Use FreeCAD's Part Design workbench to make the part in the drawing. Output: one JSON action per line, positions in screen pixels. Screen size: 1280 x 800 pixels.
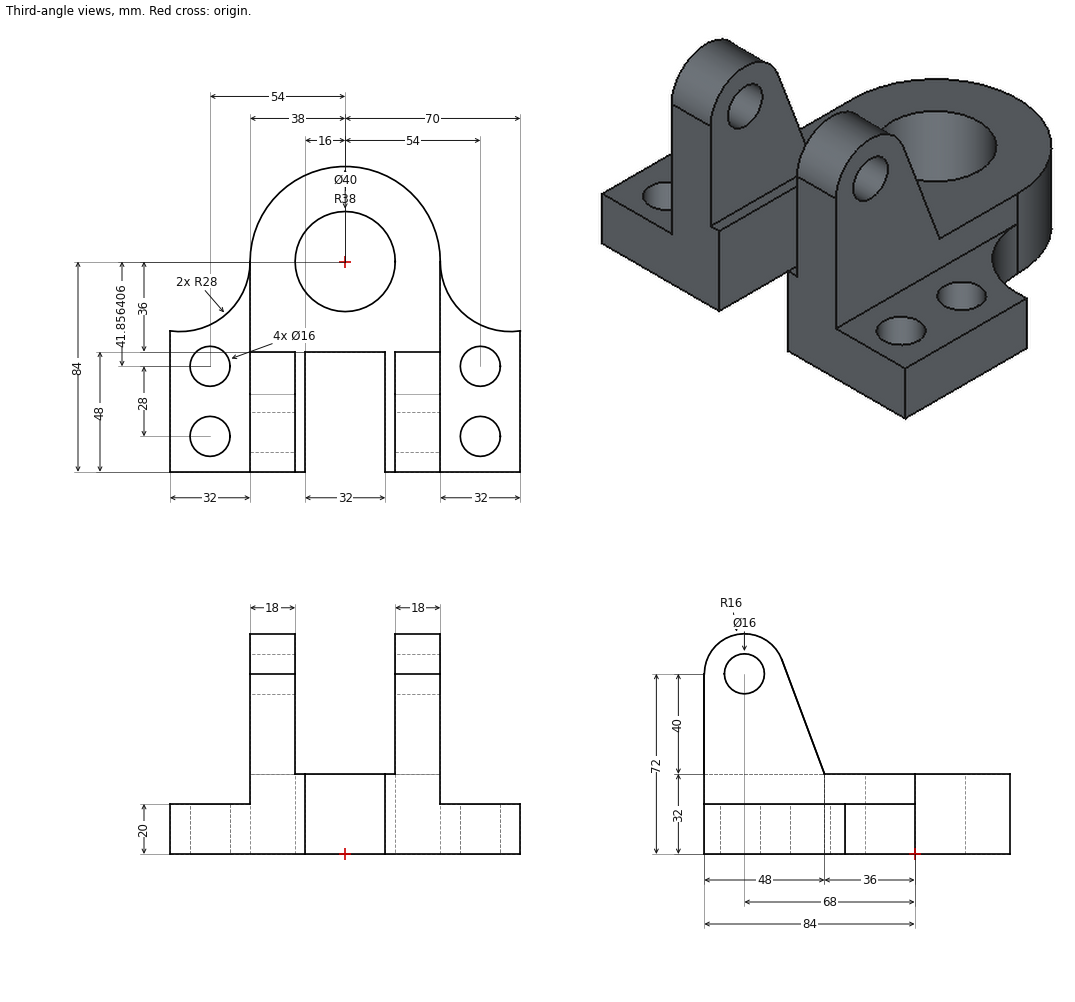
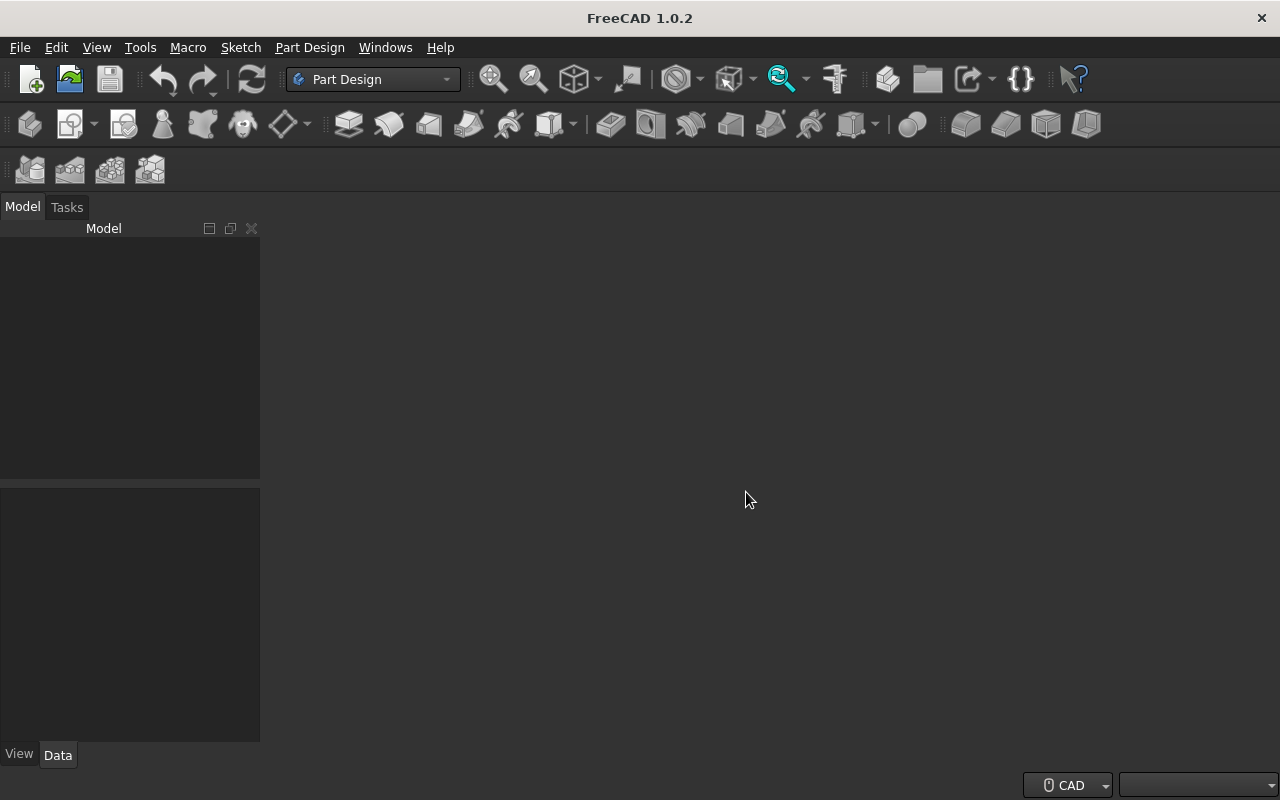
{"action": "left_click", "coordinate": [30, 80]}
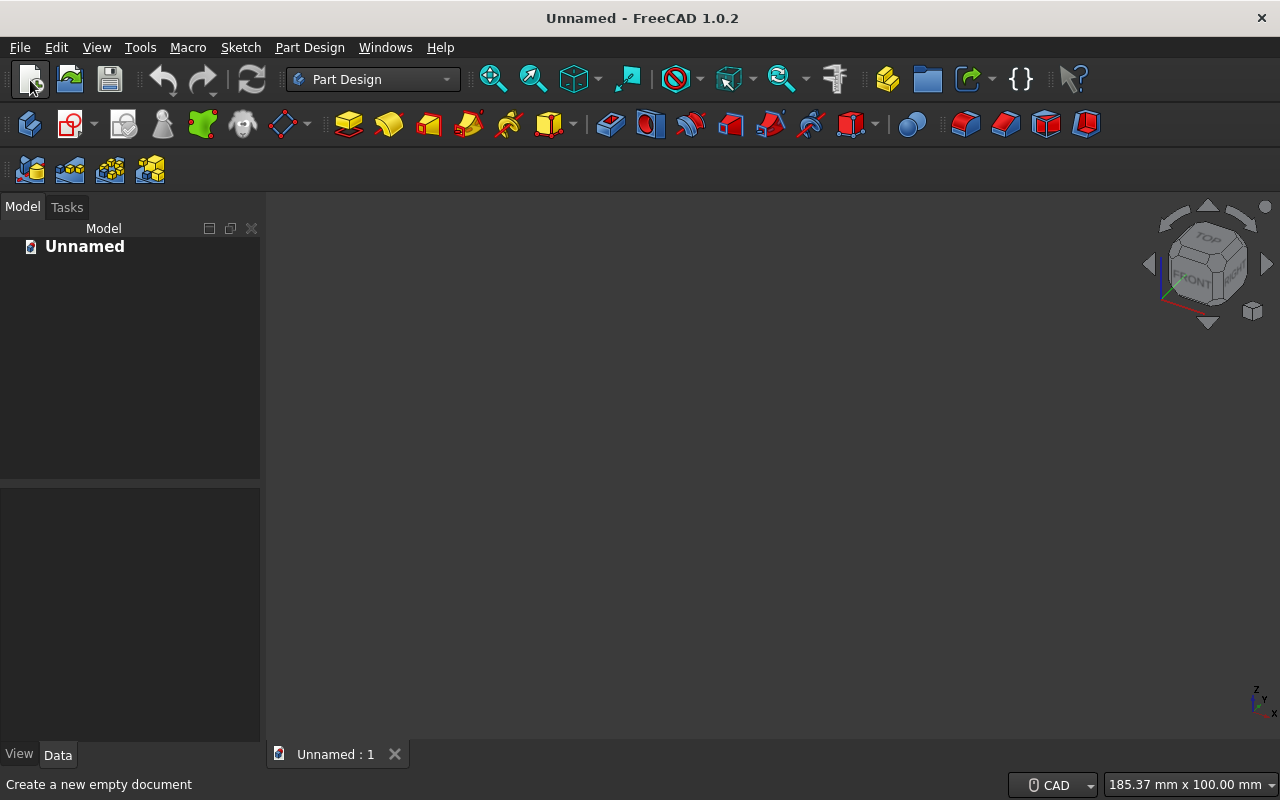
{"action": "left_click", "coordinate": [70, 124]}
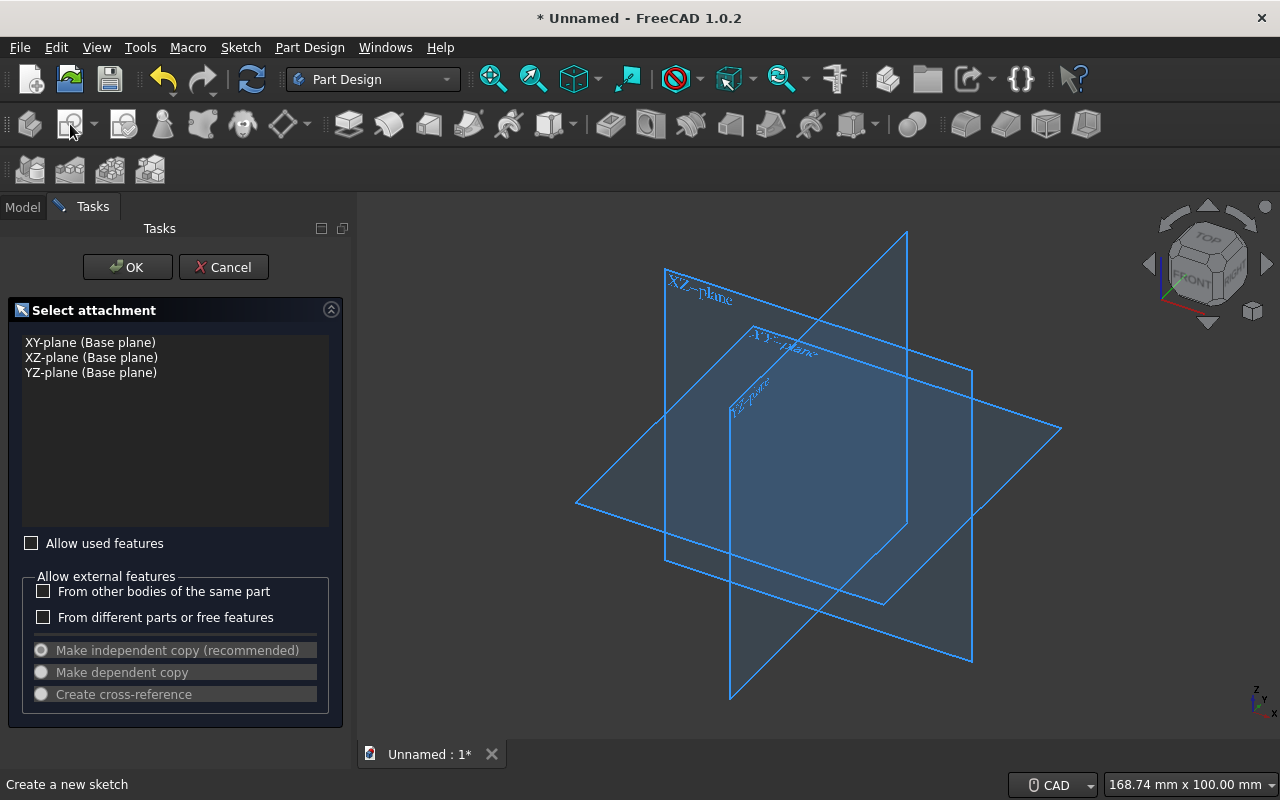
{"action": "left_click", "coordinate": [82, 342]}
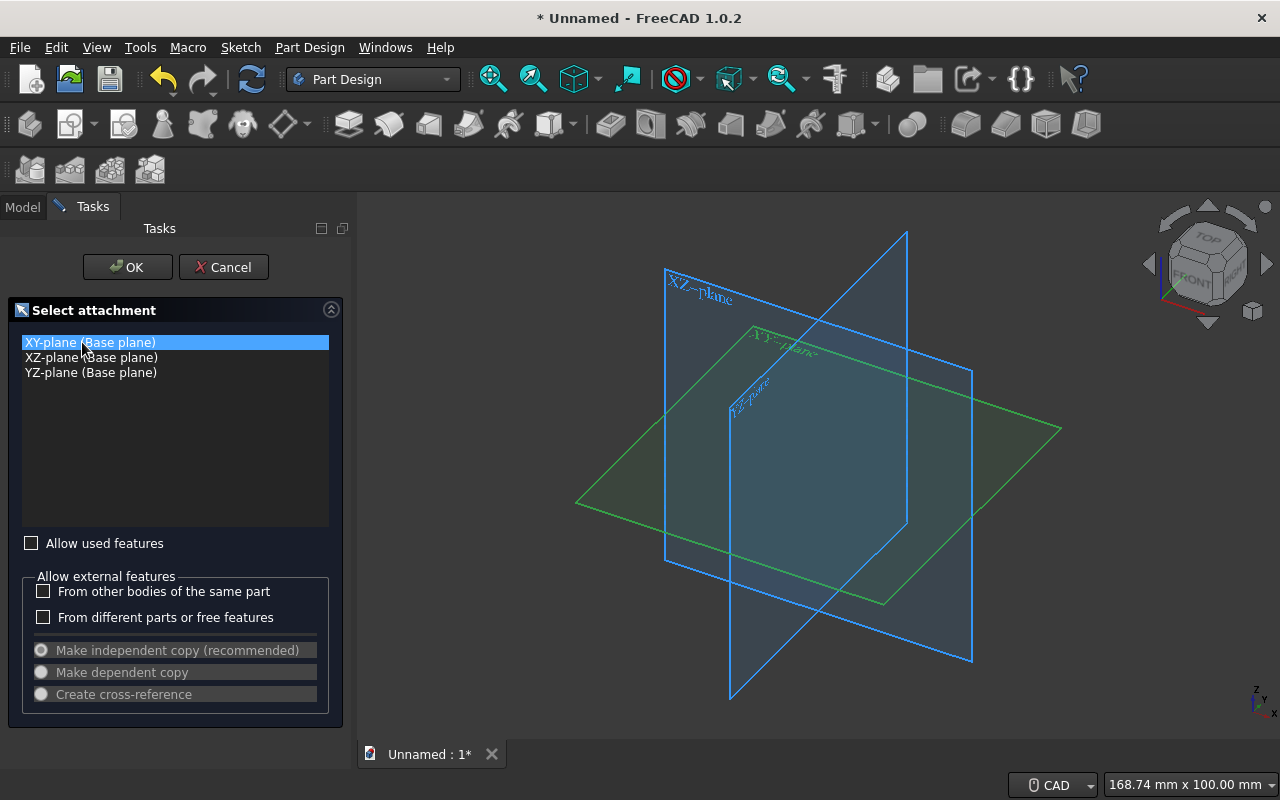
{"action": "left_click", "coordinate": [128, 267]}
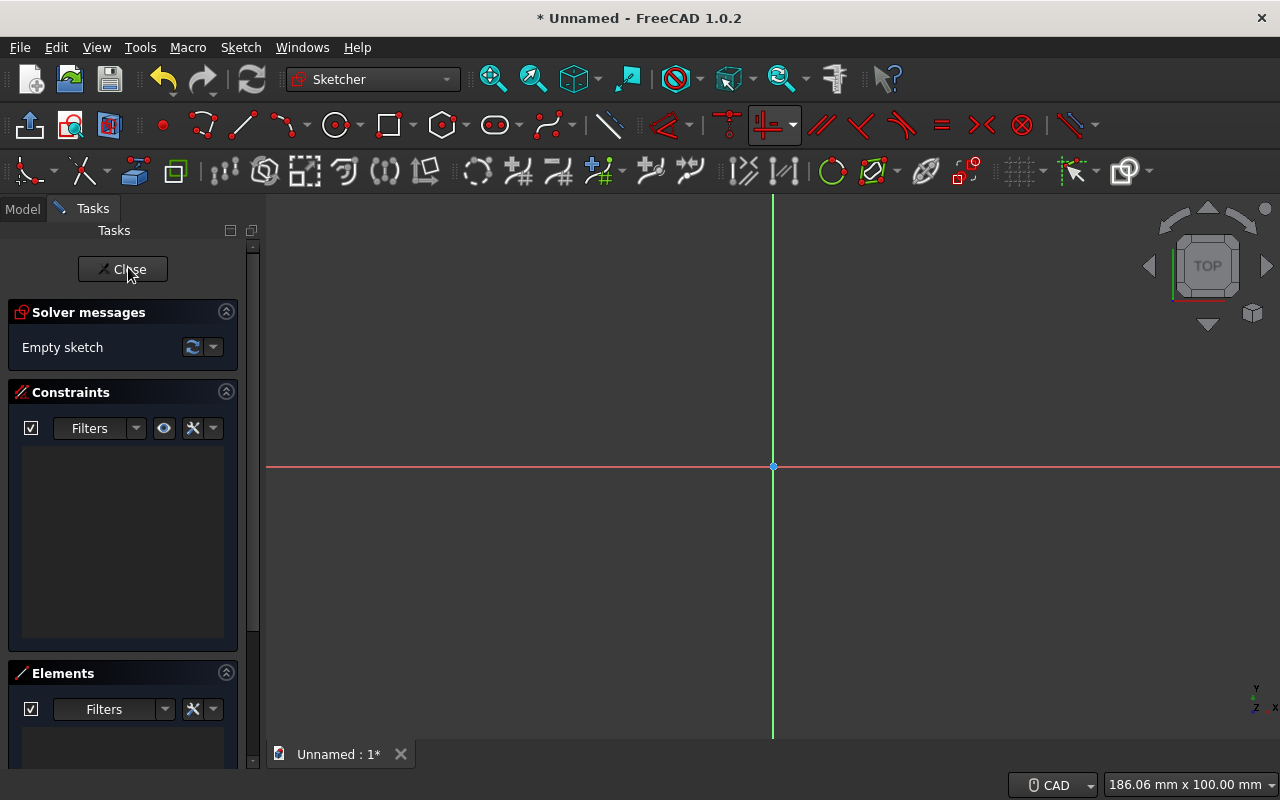
{"action": "scroll", "coordinate": [621, 314], "scroll_direction": "down", "scroll_amount": 3}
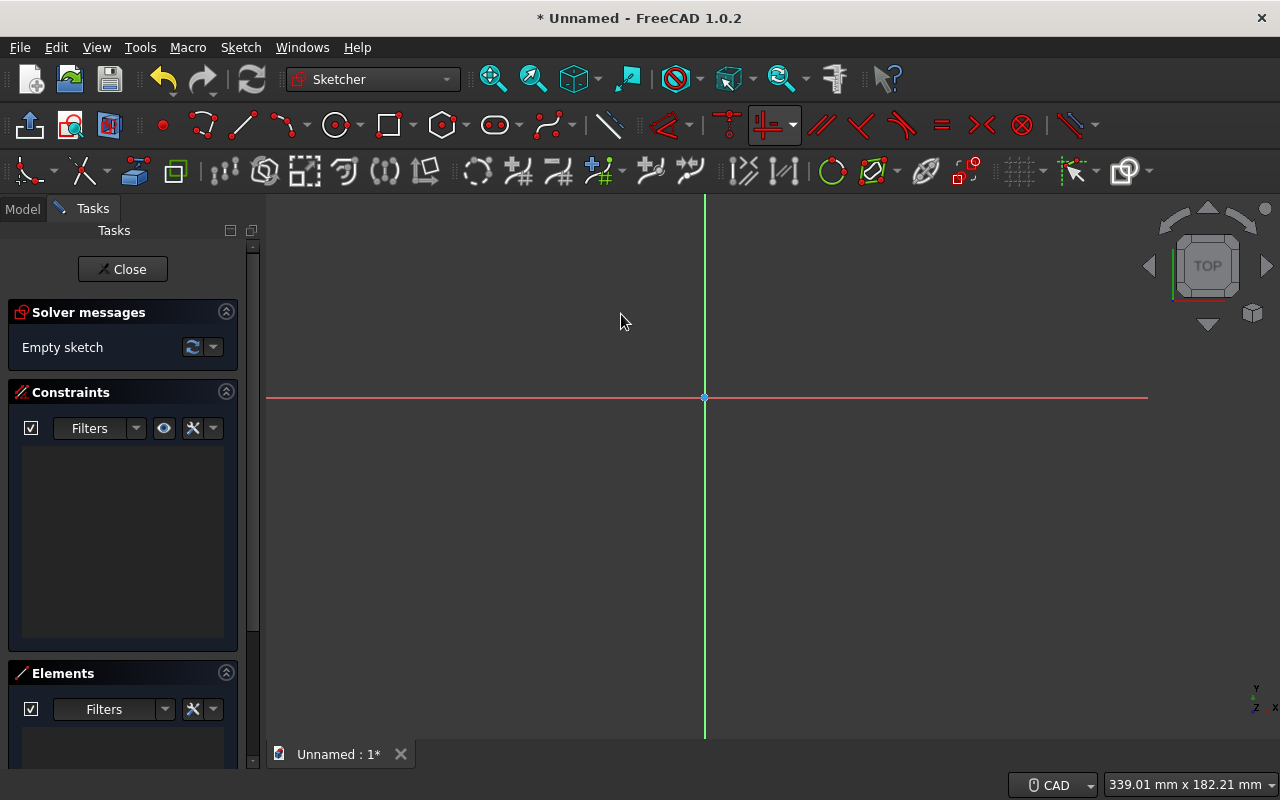
{"action": "left_click", "coordinate": [204, 126]}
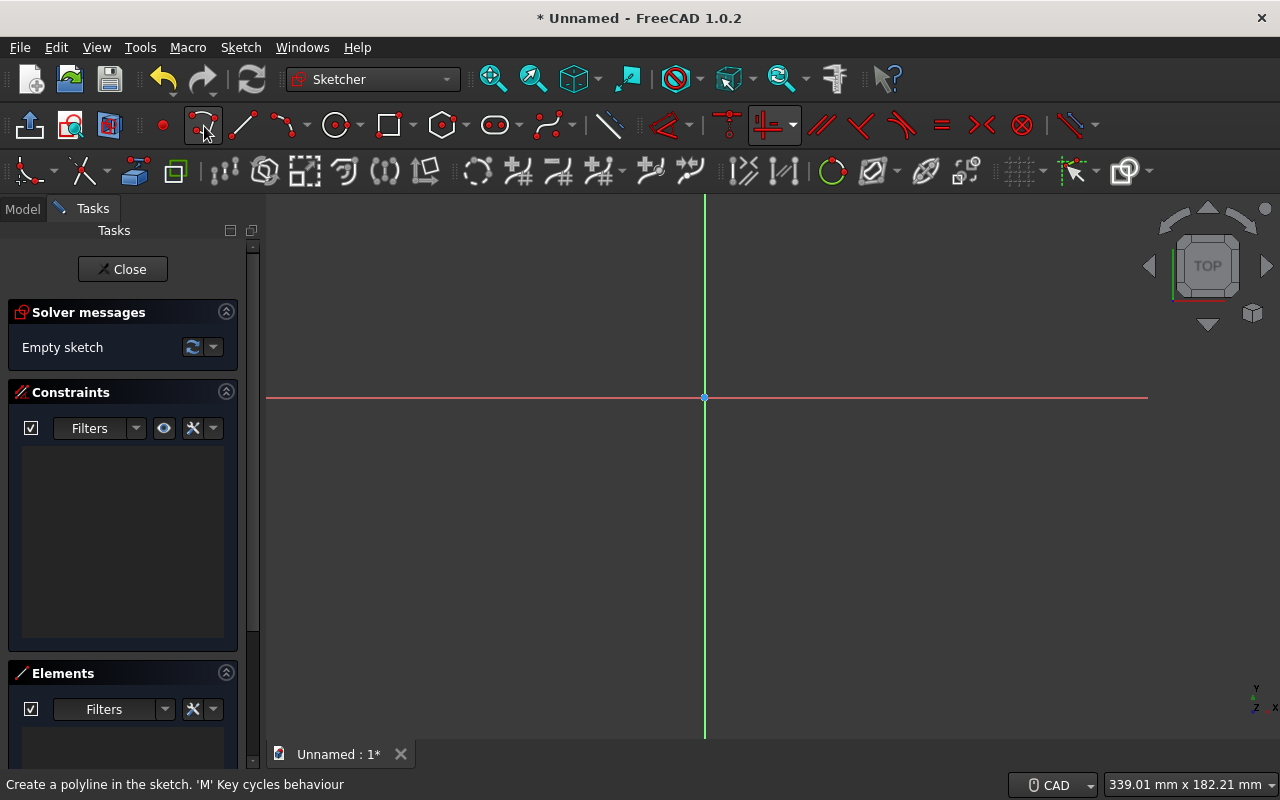
{"action": "left_click", "coordinate": [591, 398]}
{"action": "left_click", "coordinate": [591, 649]}
{"action": "left_click", "coordinate": [818, 649]}
{"action": "left_click", "coordinate": [818, 398]}
{"action": "right_click", "coordinate": [818, 398]}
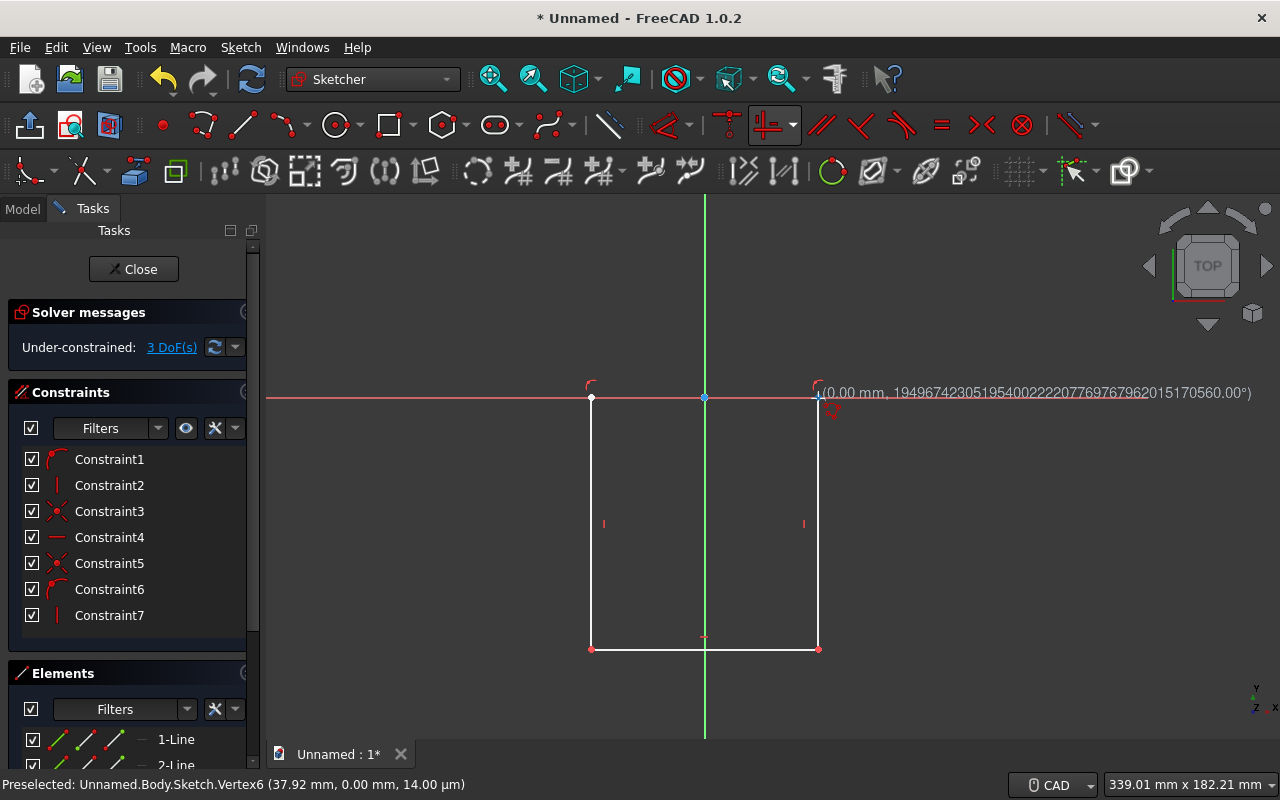
{"action": "left_click", "coordinate": [284, 126]}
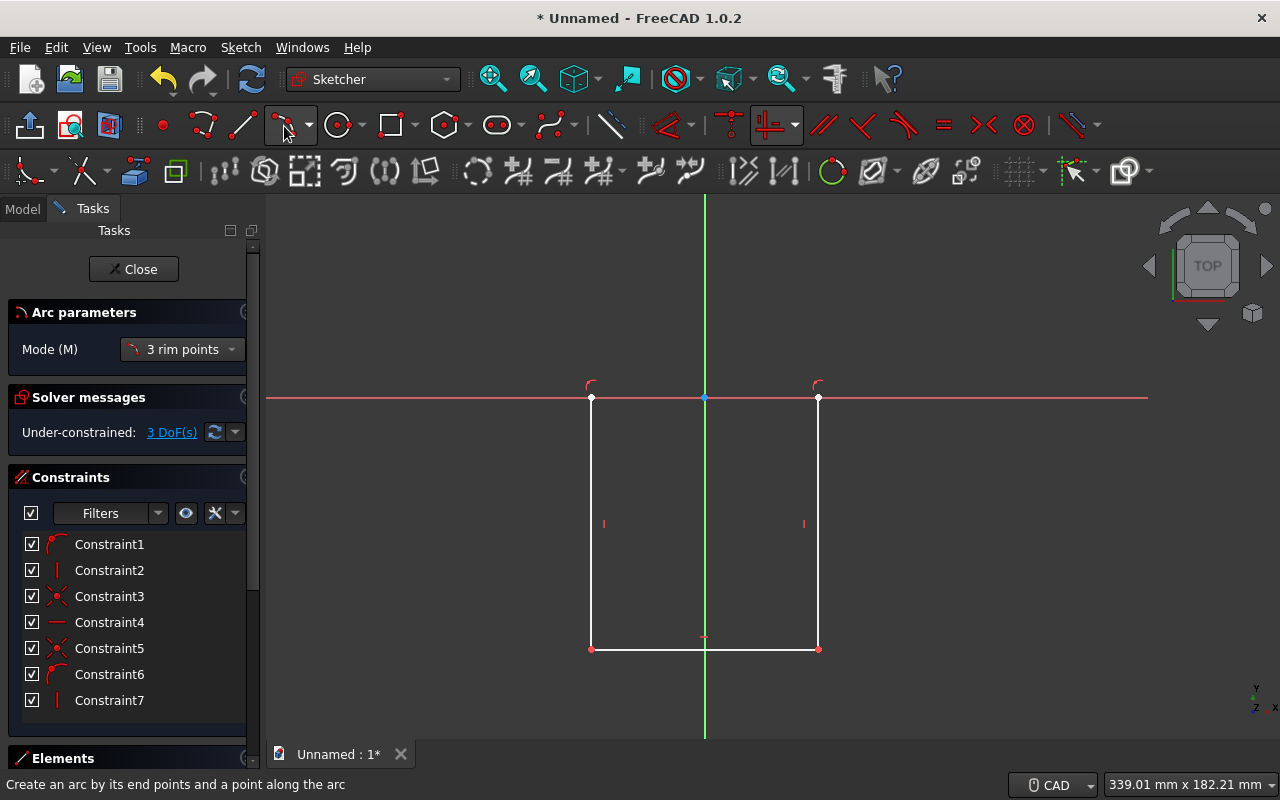
{"action": "left_click", "coordinate": [818, 398]}
{"action": "left_click", "coordinate": [591, 398]}
{"action": "left_click", "coordinate": [740, 290]}
{"action": "key", "text": "Escape"}